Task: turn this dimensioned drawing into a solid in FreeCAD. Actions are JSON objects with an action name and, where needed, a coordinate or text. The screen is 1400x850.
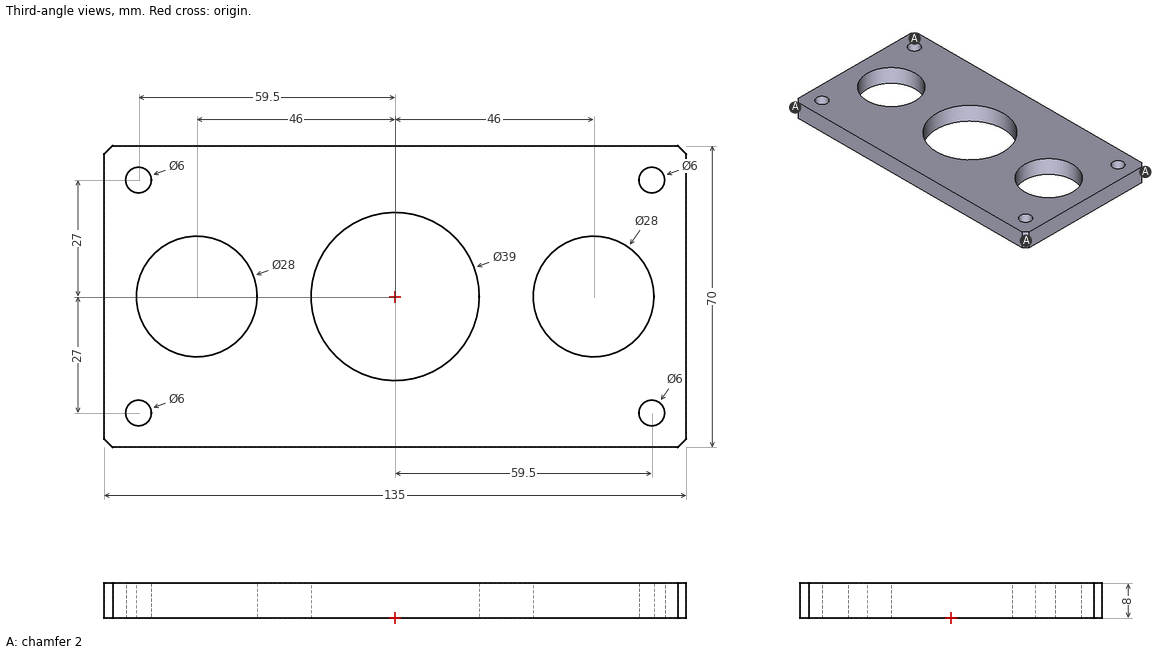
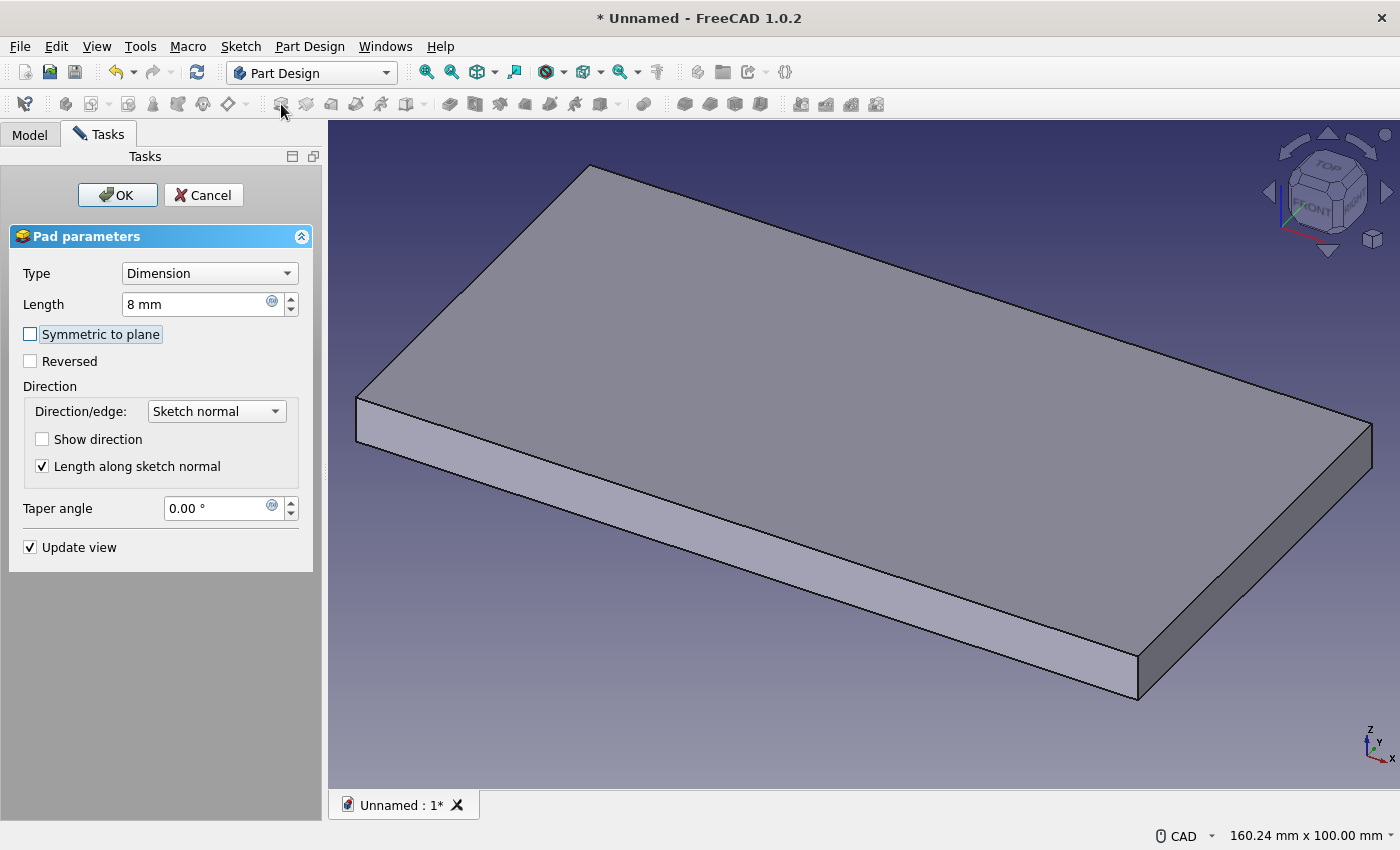
{"action": "left_click", "coordinate": [118, 195]}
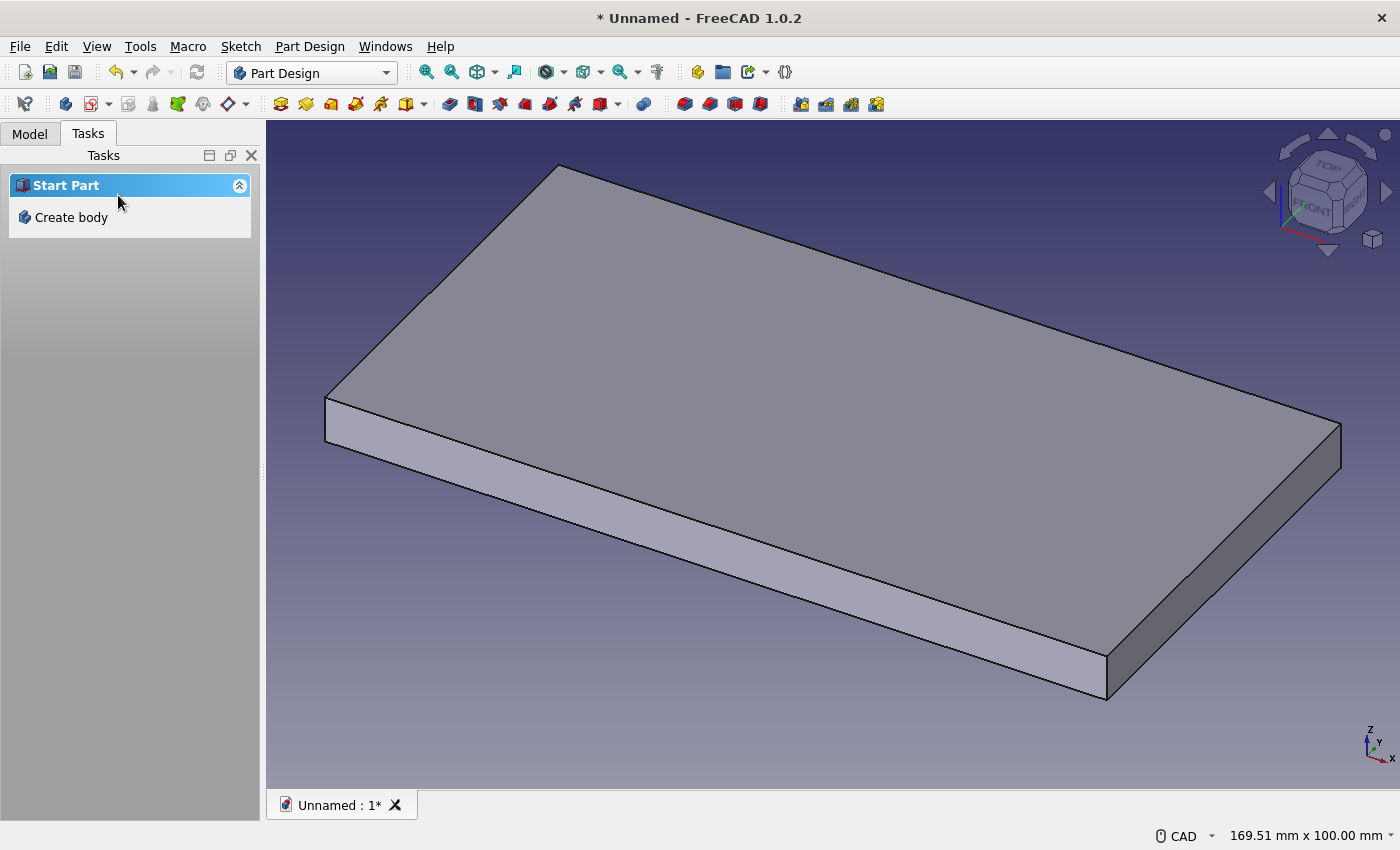
{"action": "left_click", "coordinate": [945, 447]}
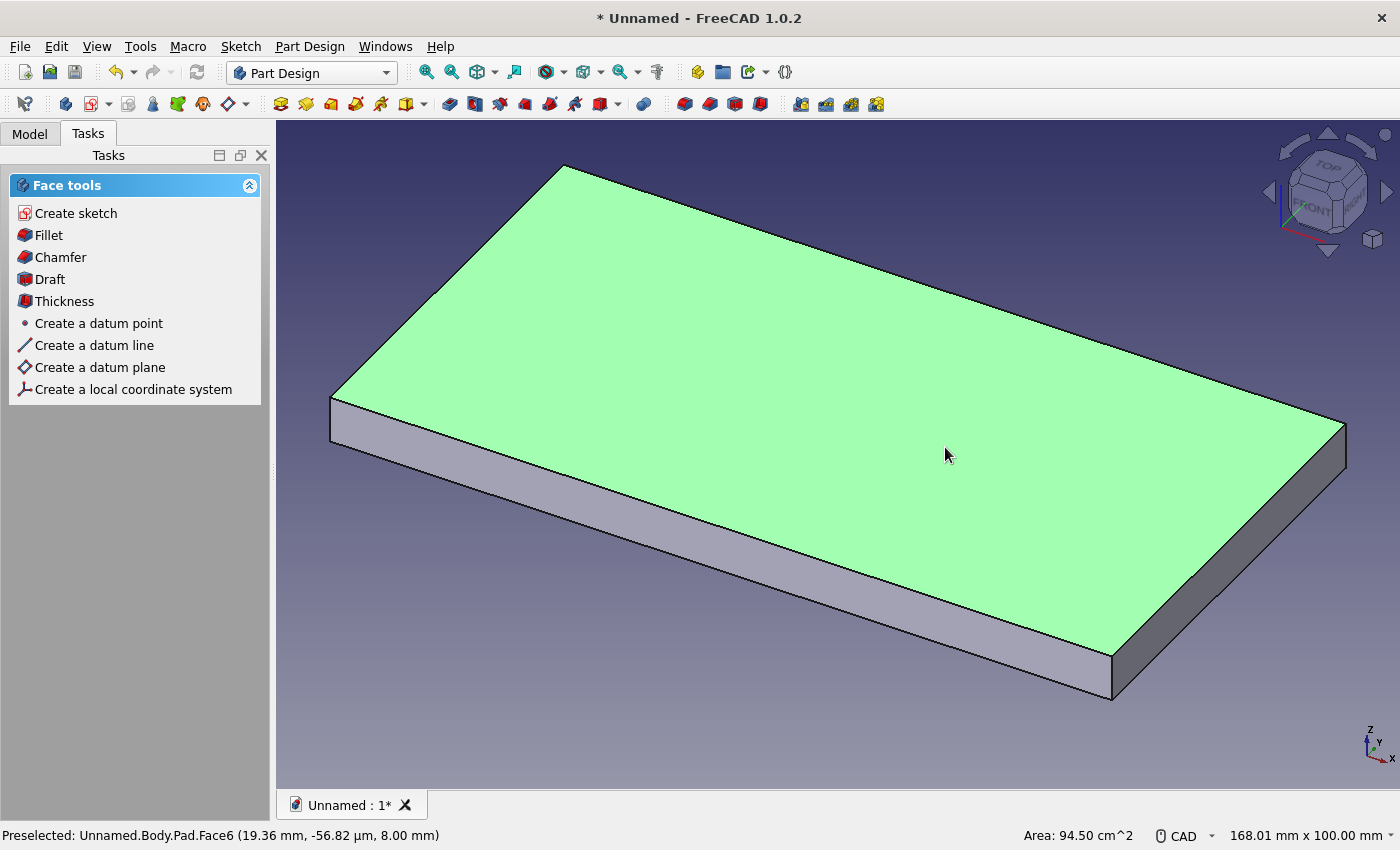
{"action": "left_click", "coordinate": [90, 104]}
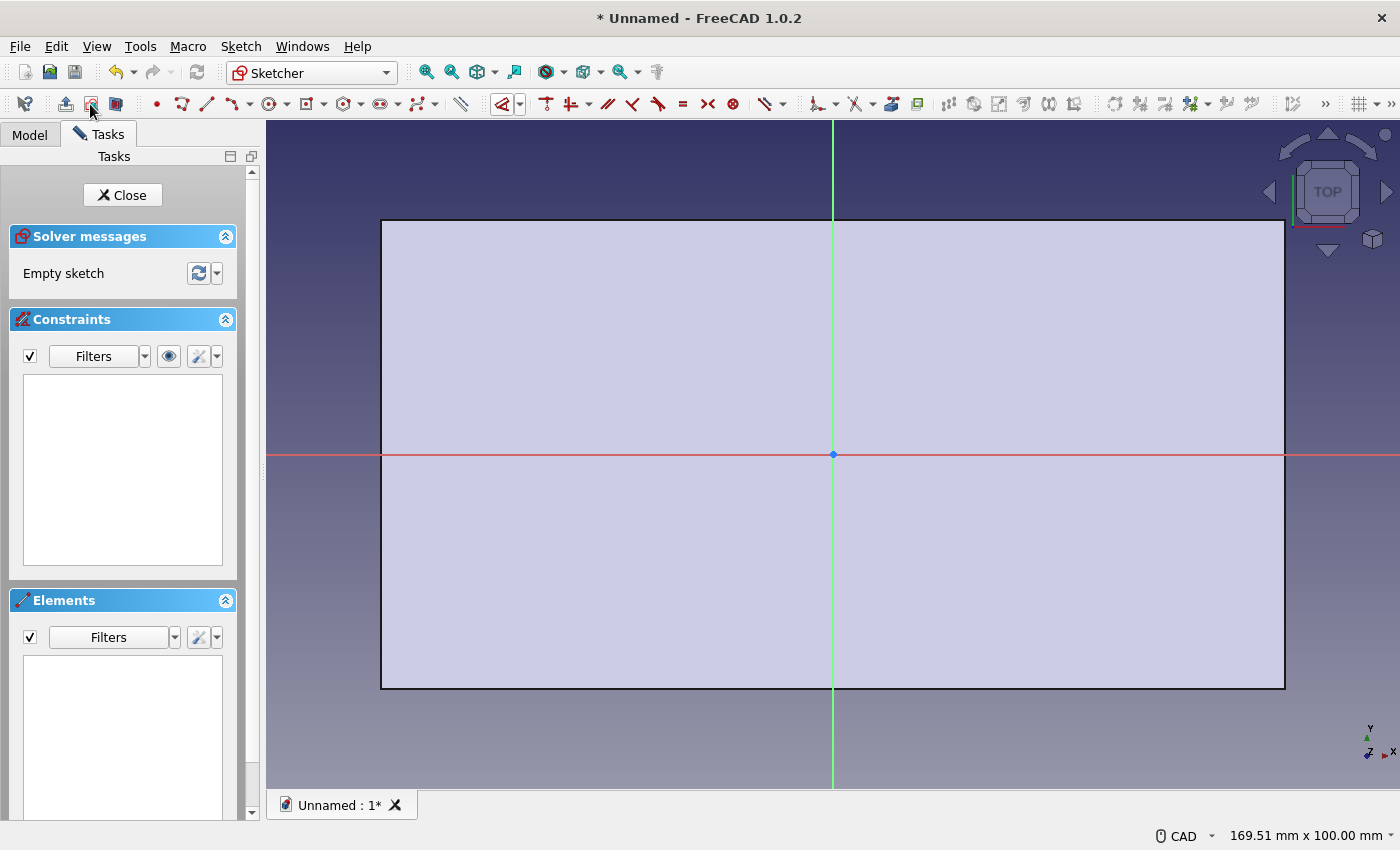
{"action": "scroll", "coordinate": [916, 454], "scroll_direction": "up", "scroll_amount": 3}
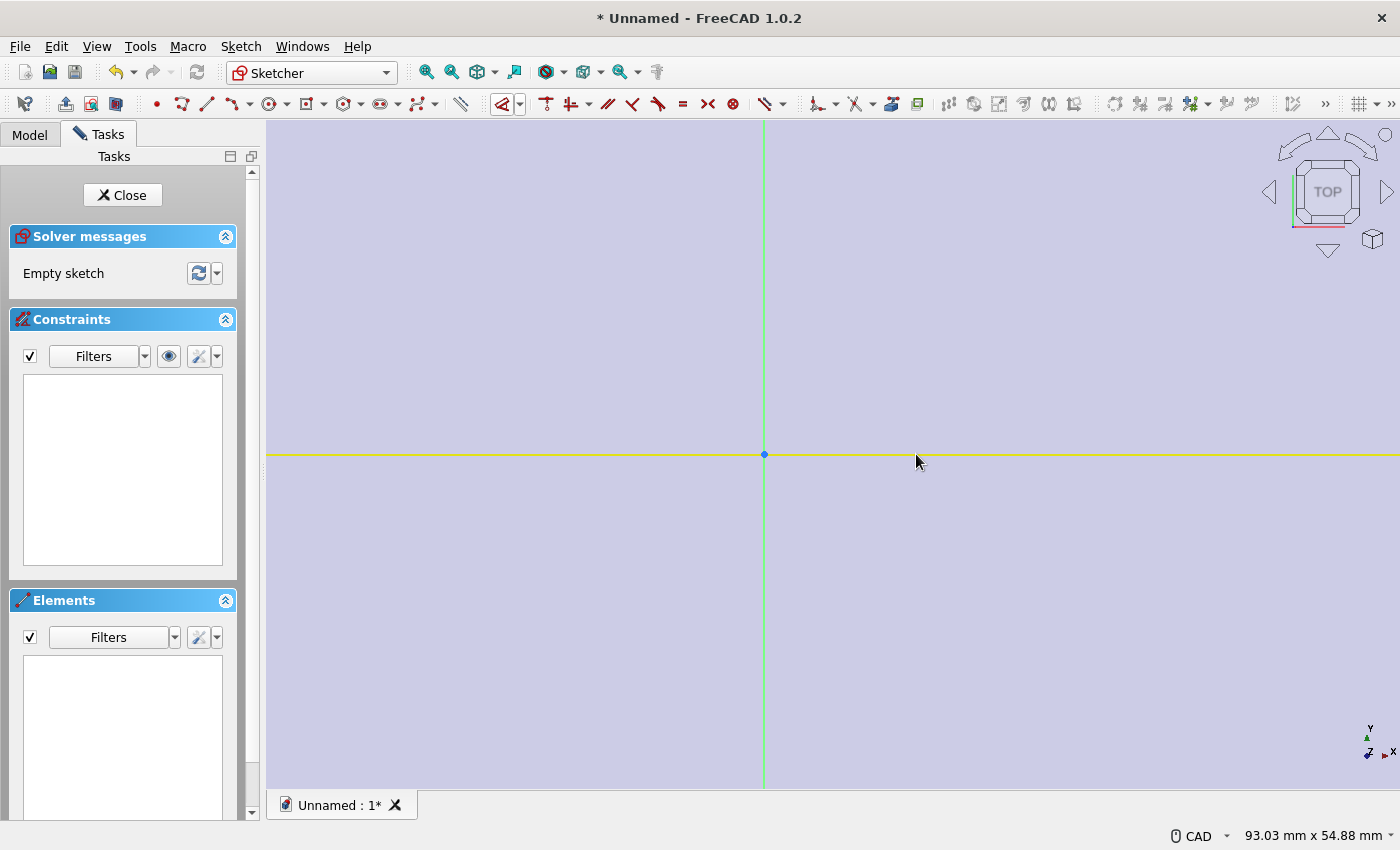
{"action": "key", "text": "g c"}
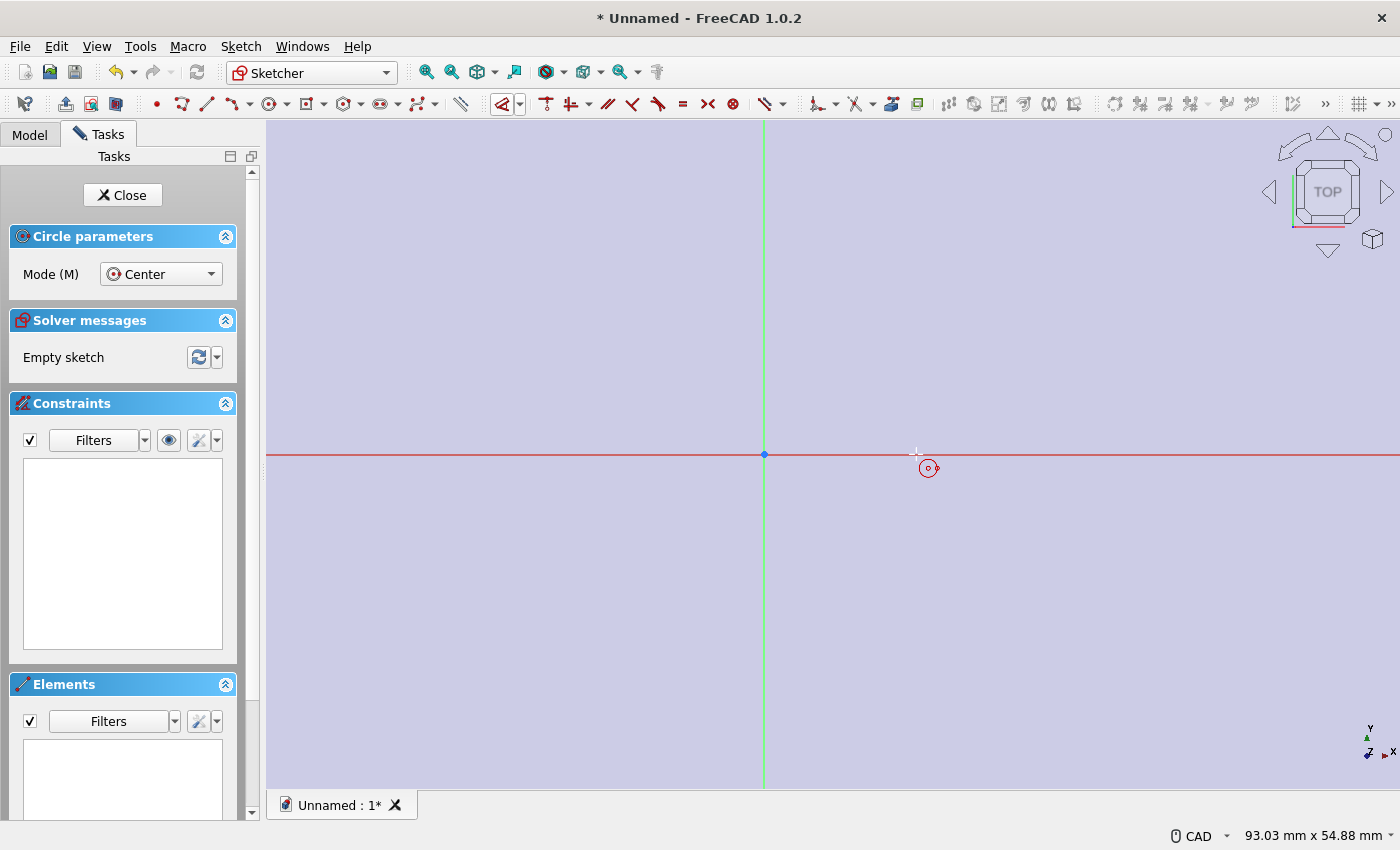
{"action": "left_click", "coordinate": [764, 454]}
{"action": "left_click", "coordinate": [932, 286]}
{"action": "key", "text": "Escape"}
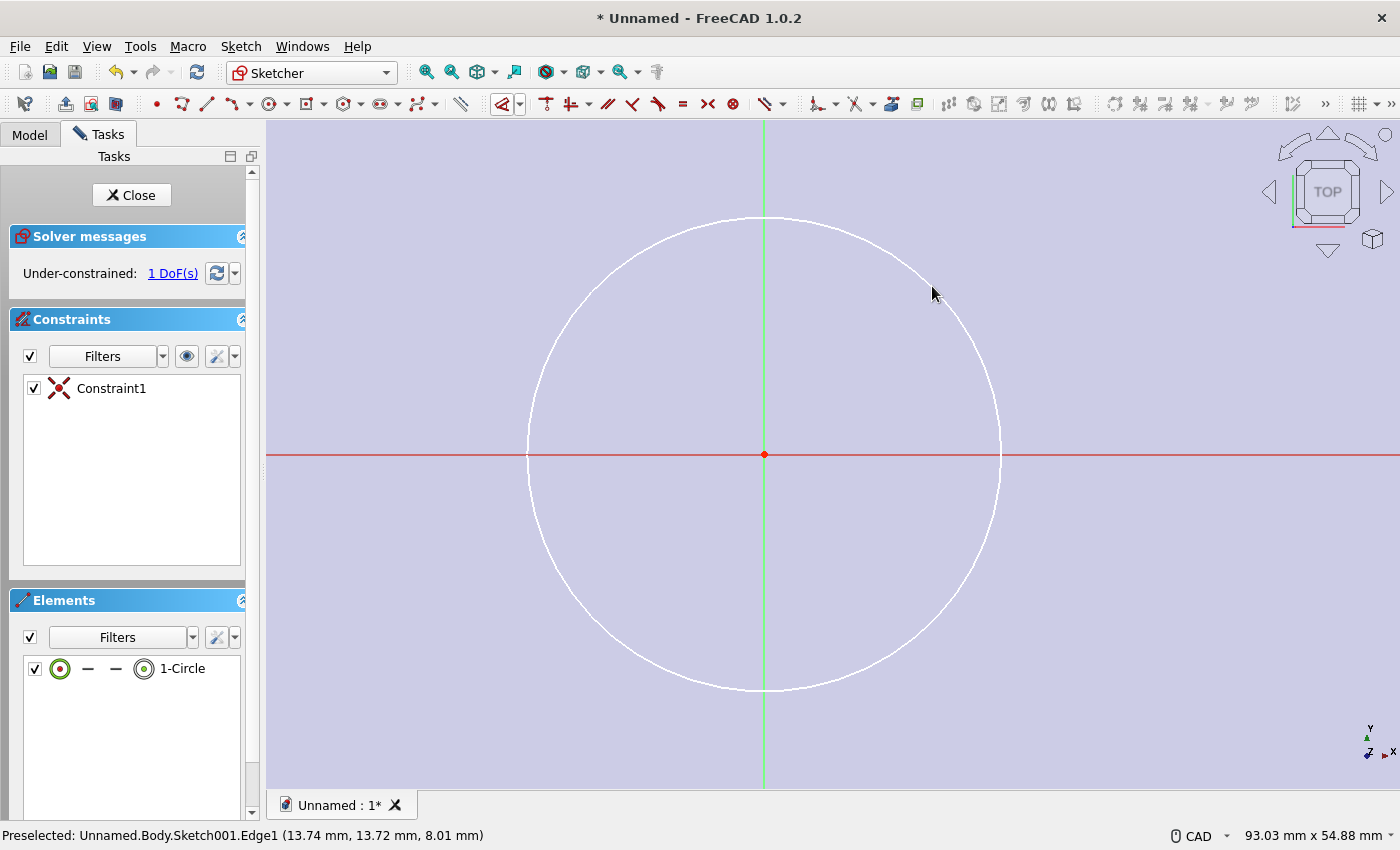
{"action": "left_click", "coordinate": [931, 286]}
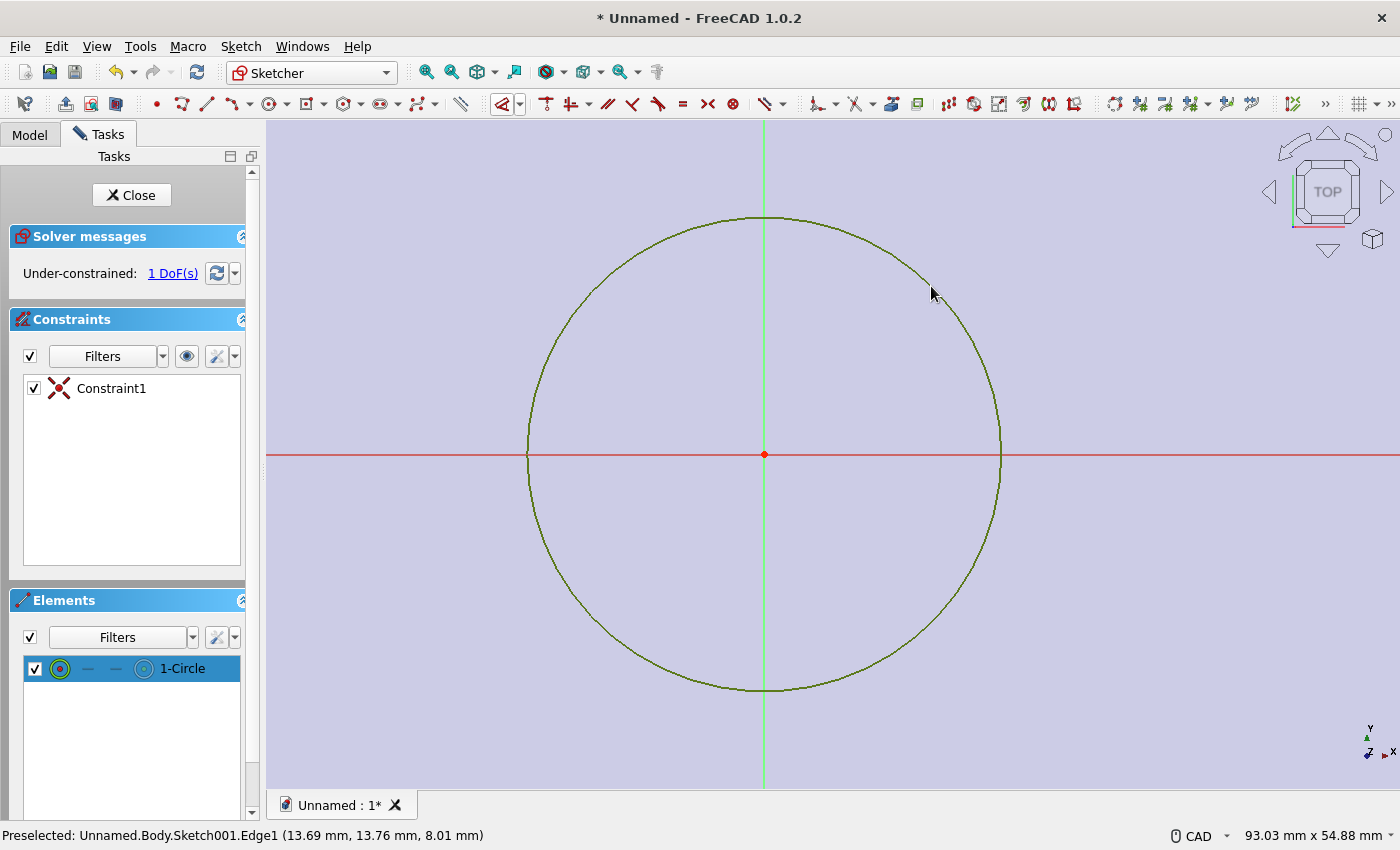
{"action": "key", "text": "k o"}